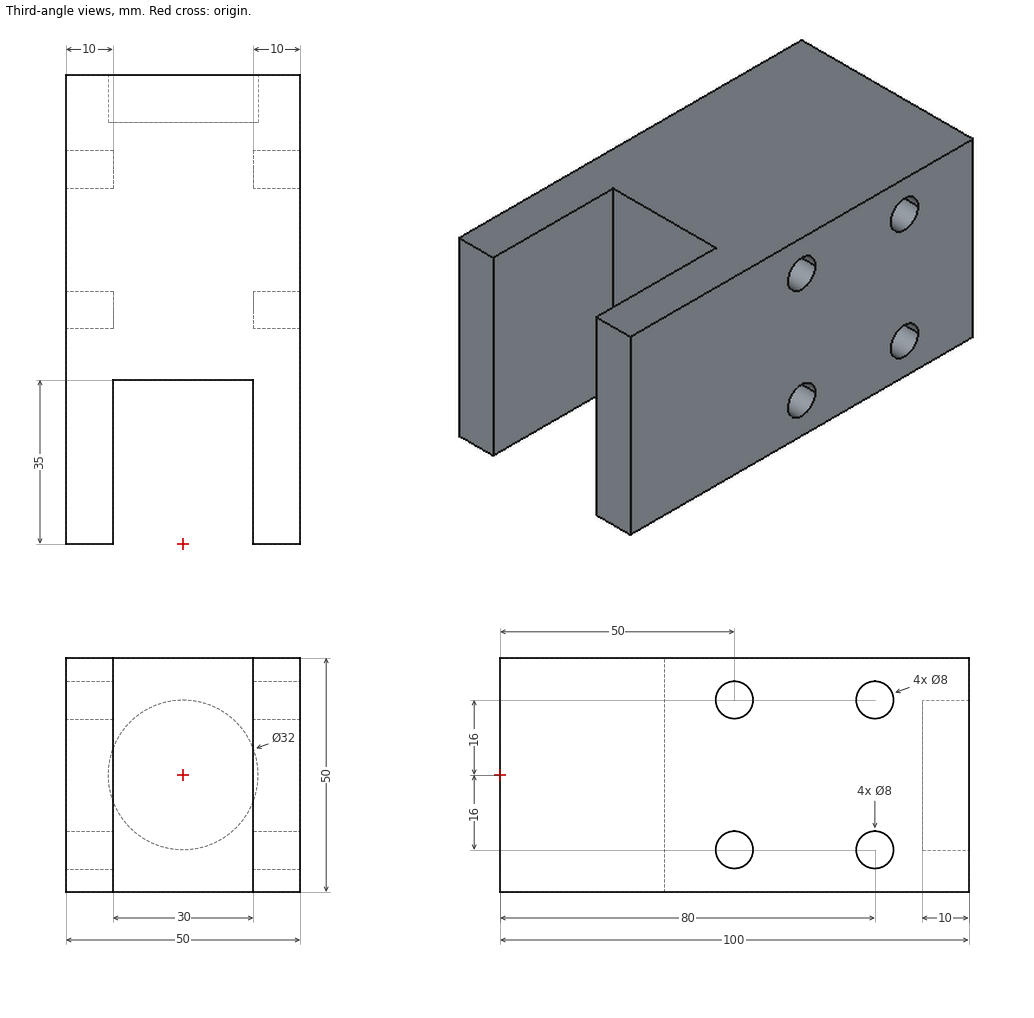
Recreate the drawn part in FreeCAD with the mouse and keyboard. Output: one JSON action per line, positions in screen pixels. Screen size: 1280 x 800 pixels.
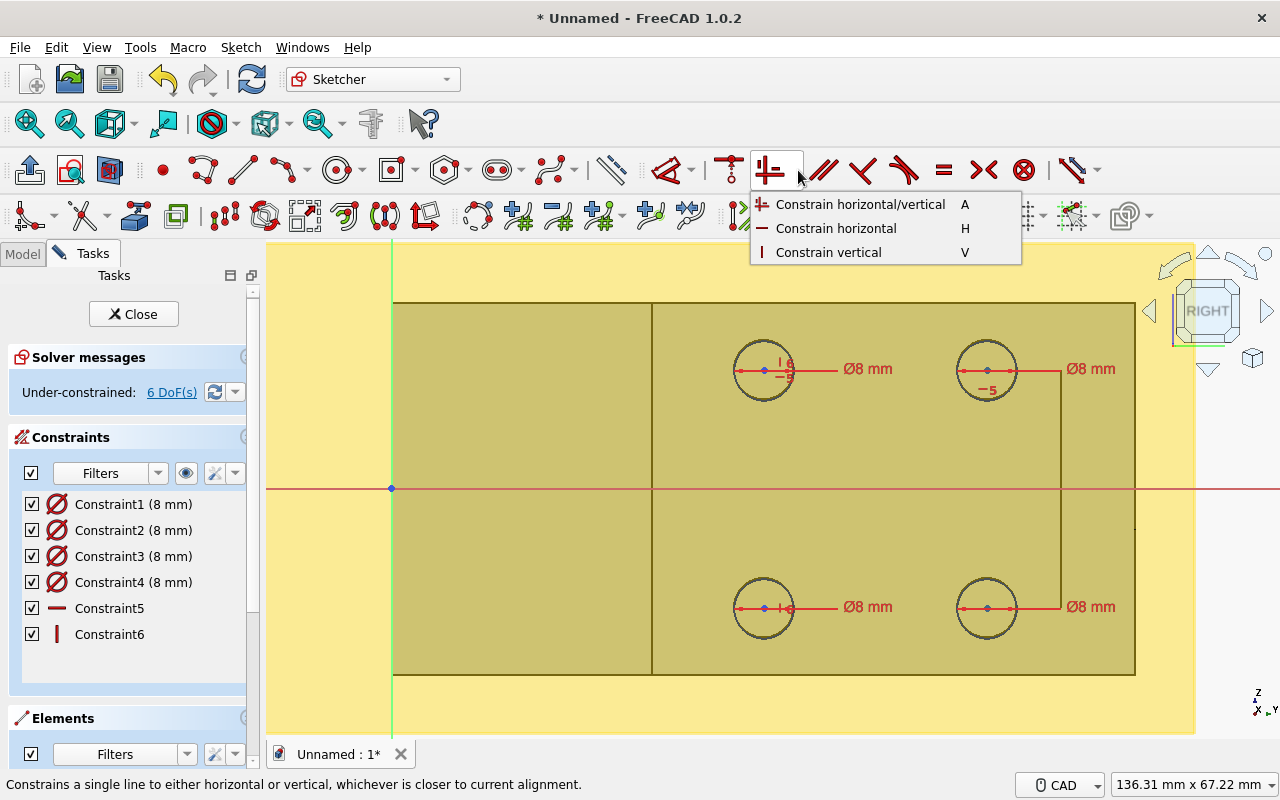
{"action": "left_click", "coordinate": [886, 252]}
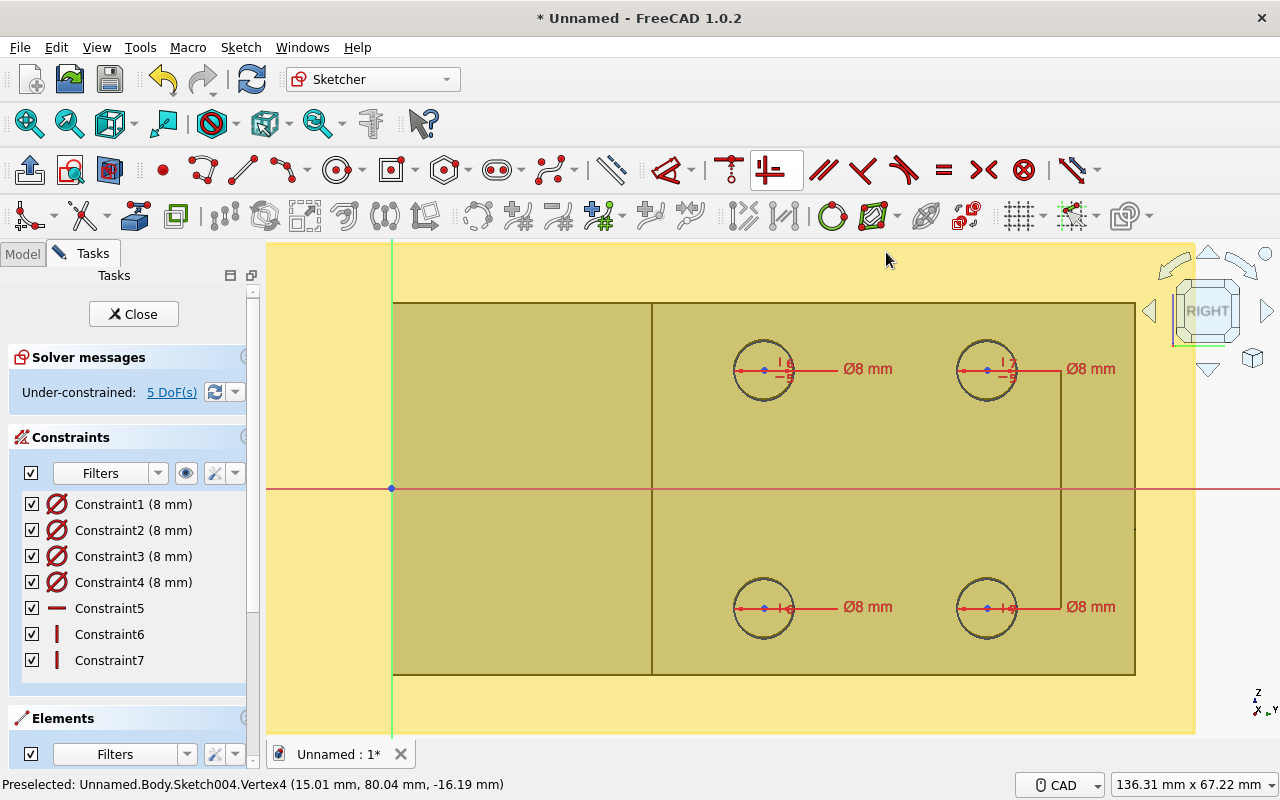
{"action": "left_click", "coordinate": [764, 609]}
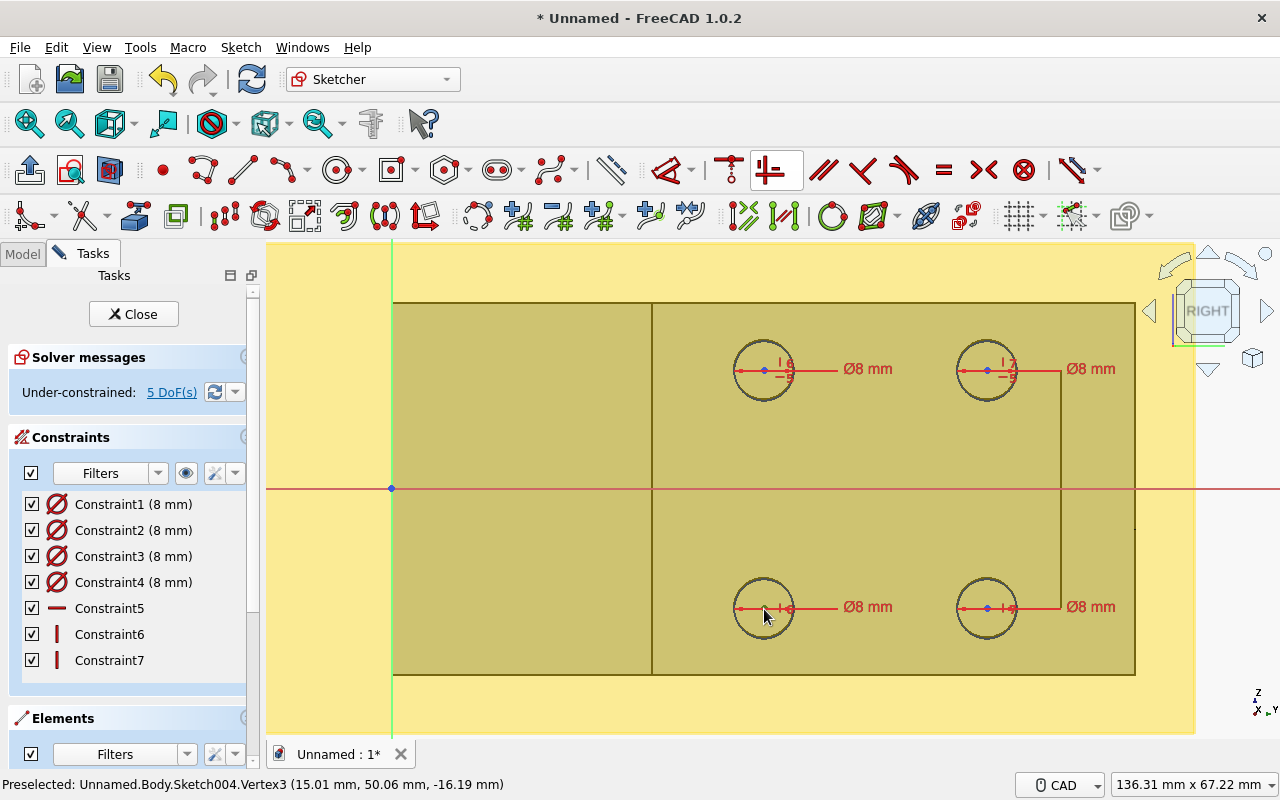
{"action": "left_click", "coordinate": [987, 609]}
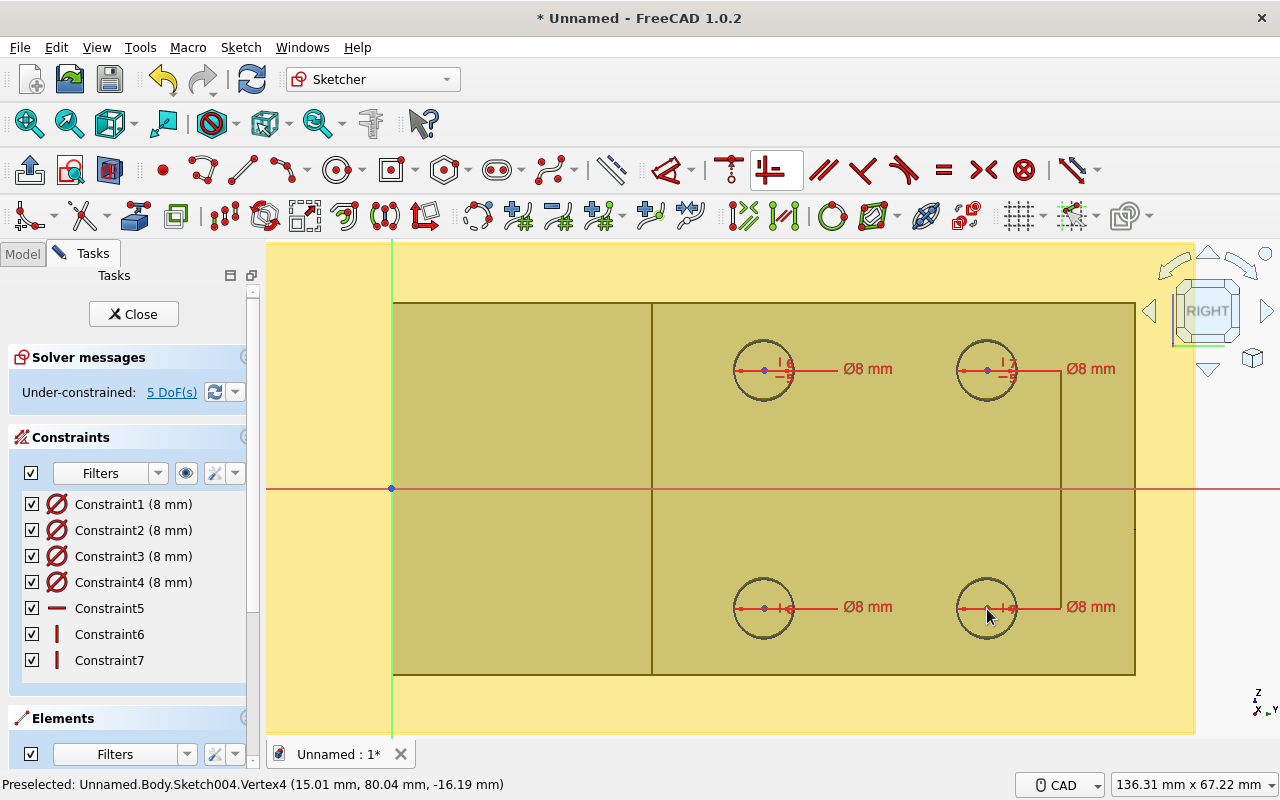
{"action": "left_click", "coordinate": [798, 170]}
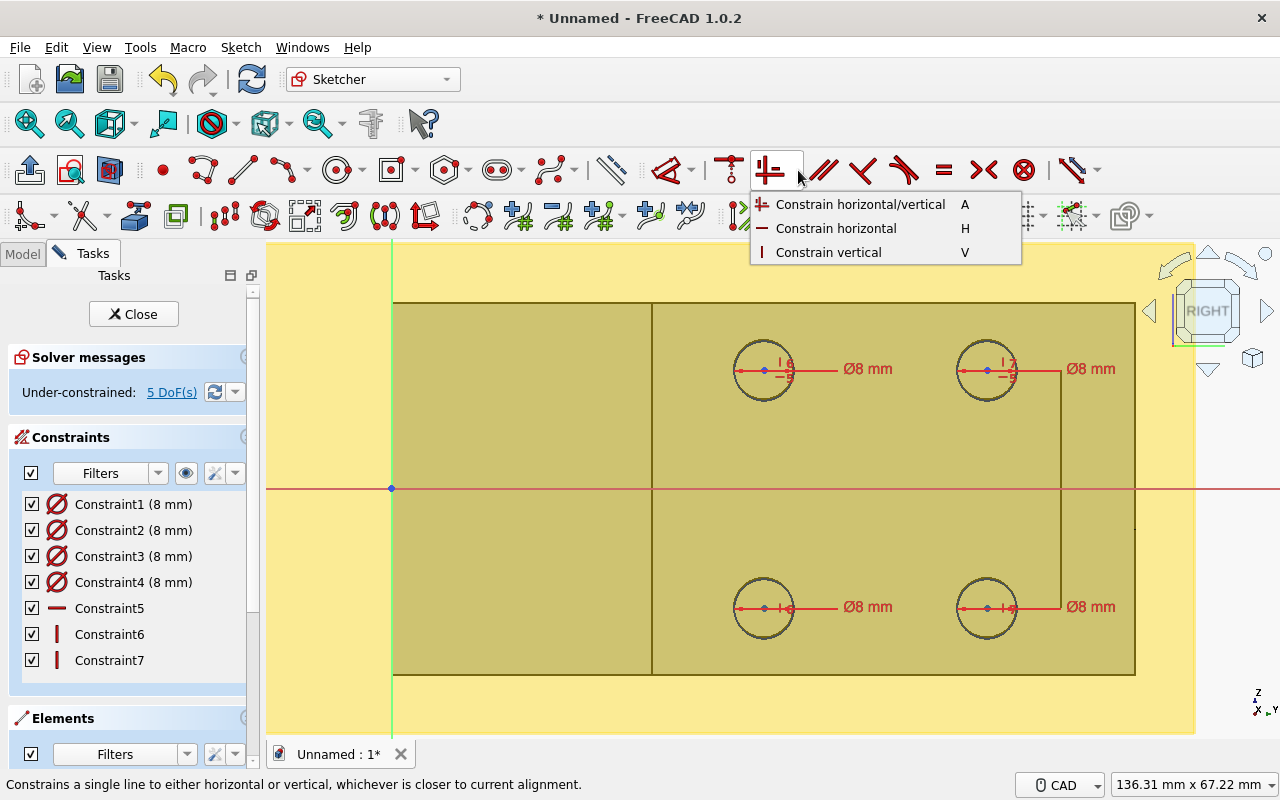
{"action": "left_click", "coordinate": [886, 228]}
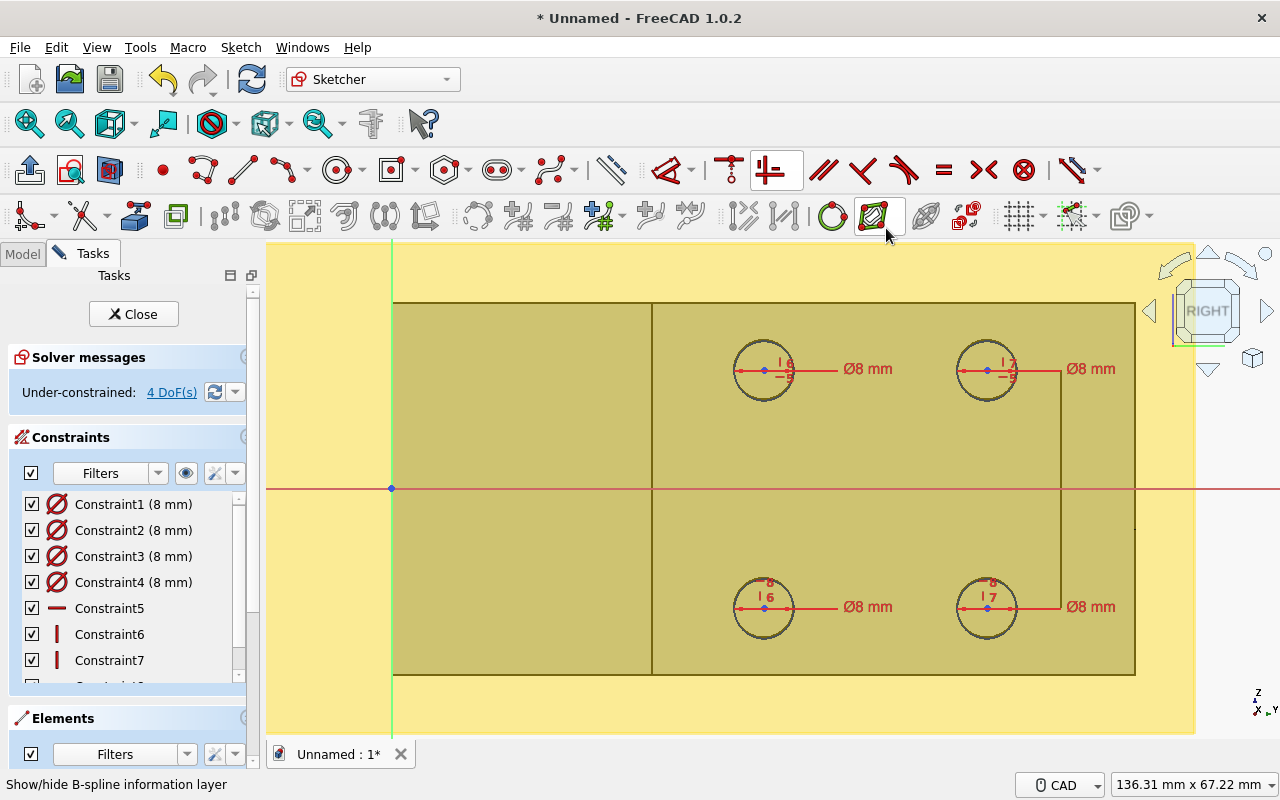
{"action": "left_click", "coordinate": [666, 170]}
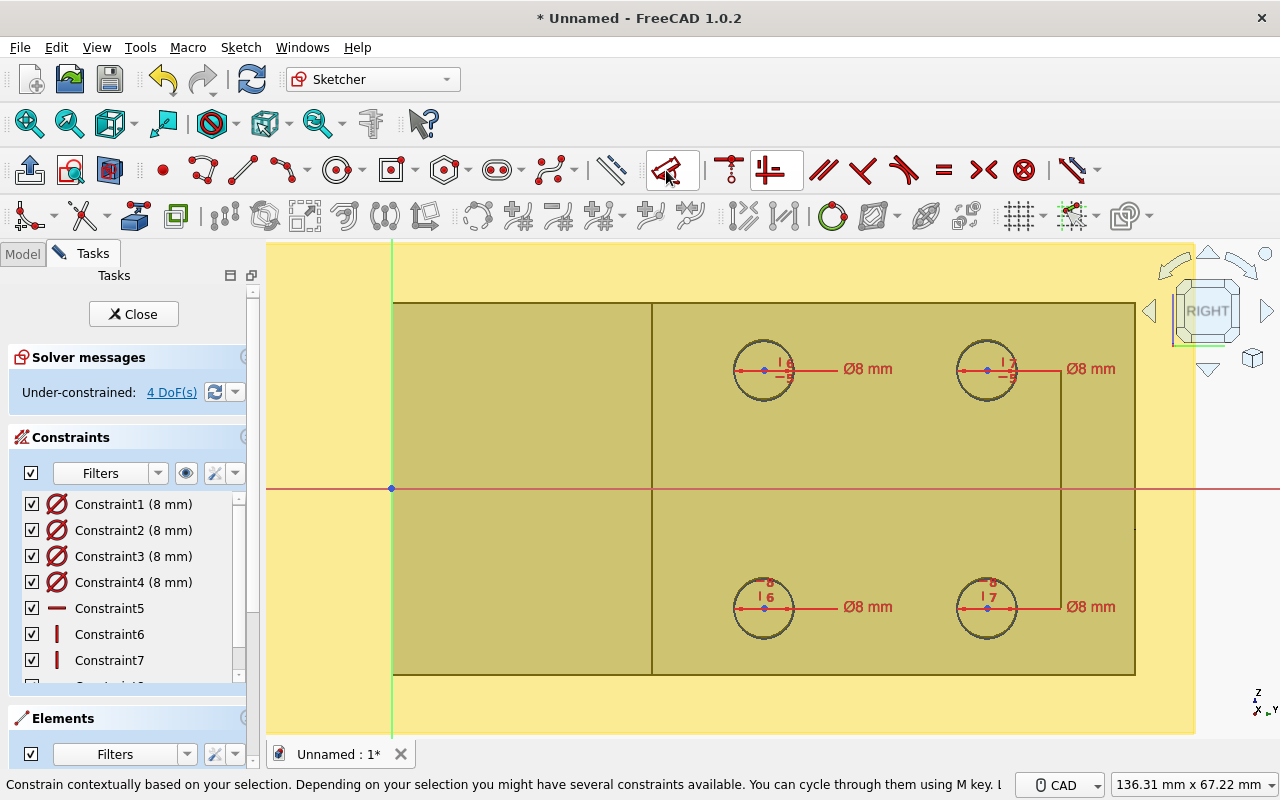
{"action": "left_click", "coordinate": [987, 371]}
{"action": "left_click", "coordinate": [689, 337]}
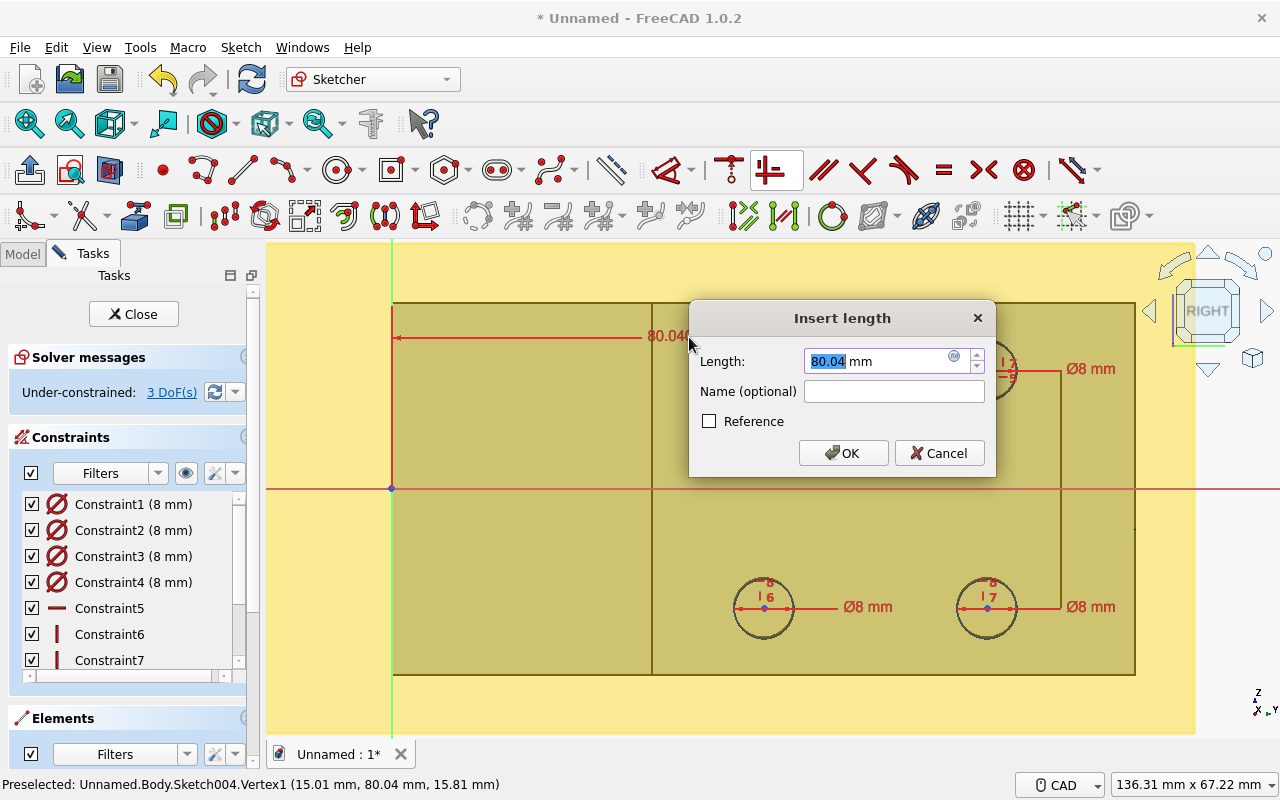
{"action": "type", "text": "80"}
{"action": "key", "text": "Return"}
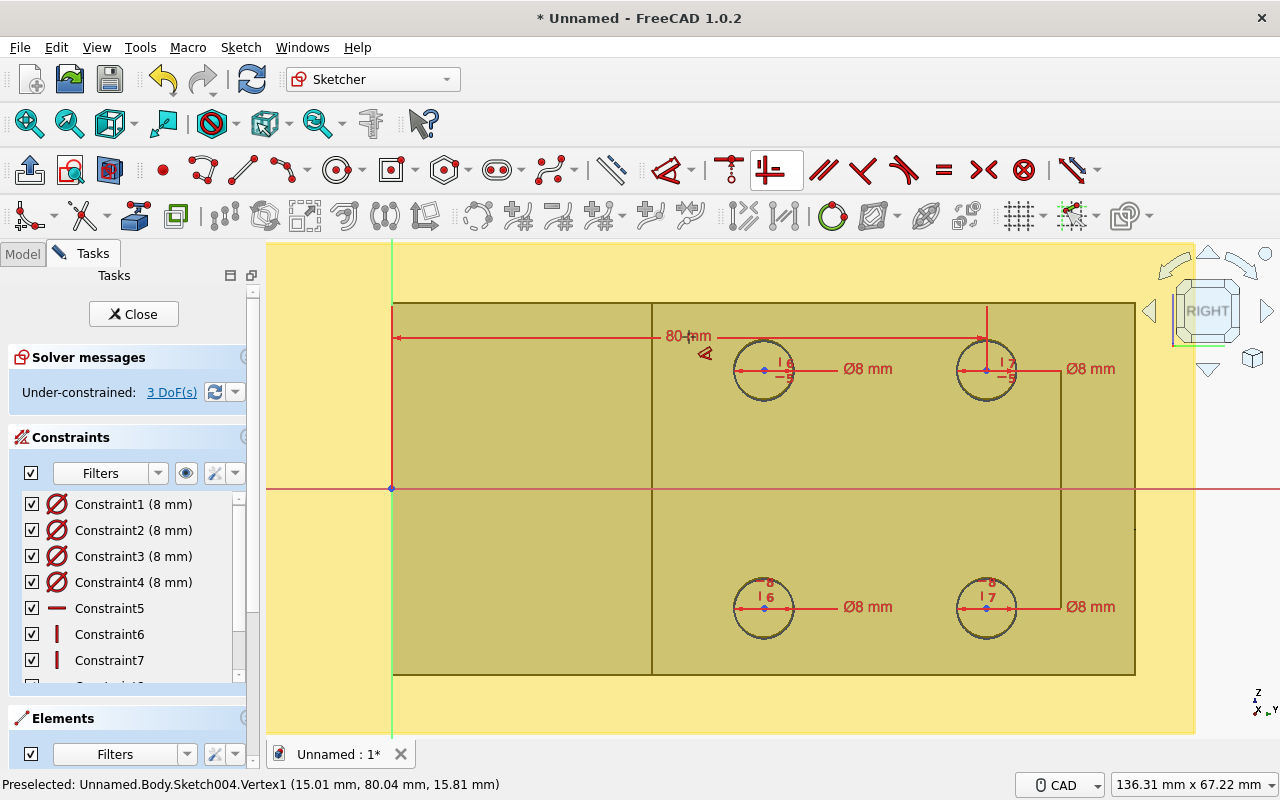
{"action": "left_click", "coordinate": [987, 371]}
{"action": "left_click", "coordinate": [358, 430]}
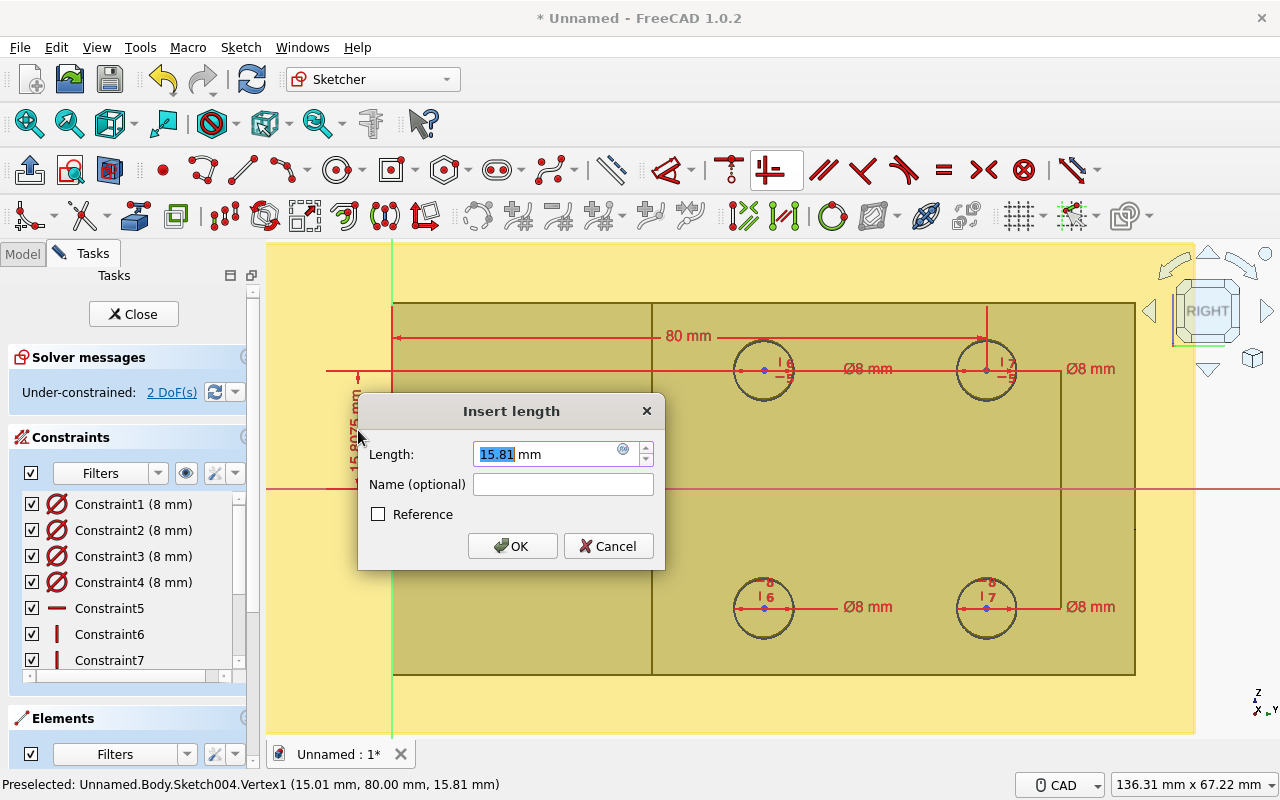
{"action": "type", "text": "16"}
{"action": "key", "text": "Return"}